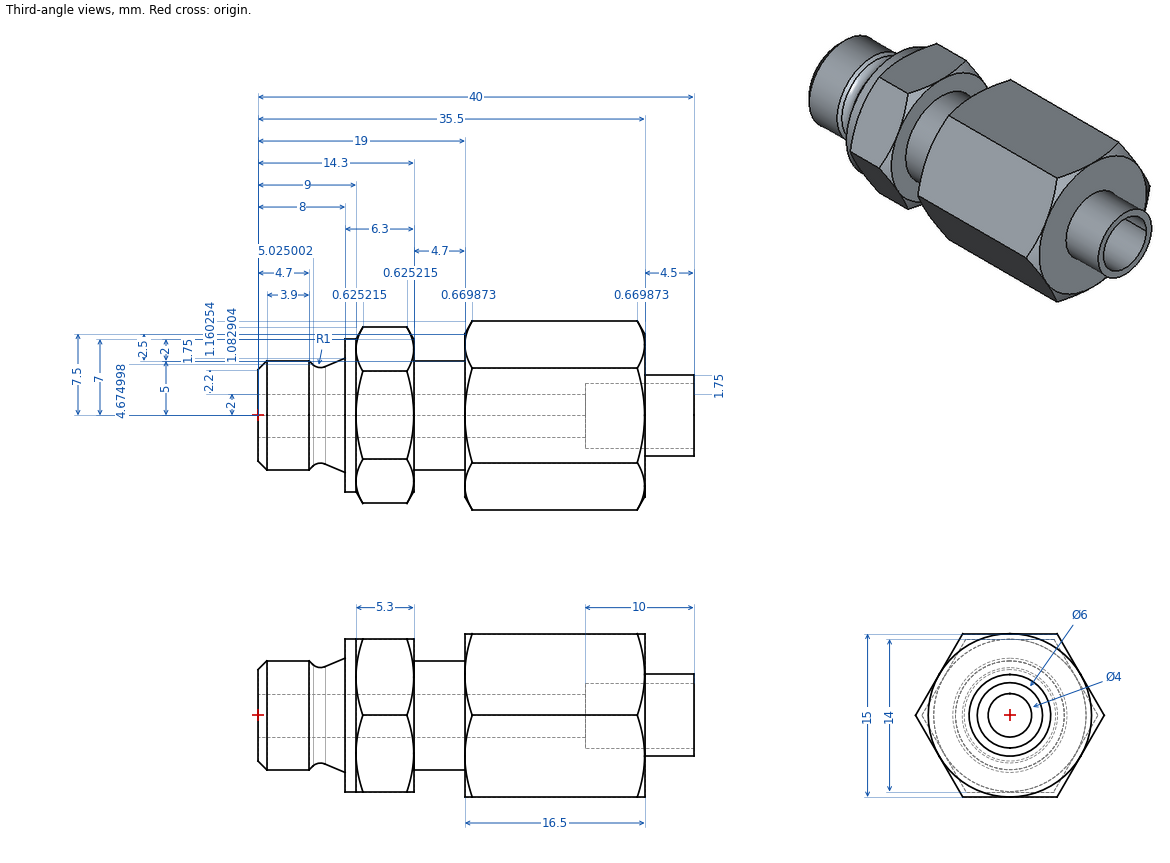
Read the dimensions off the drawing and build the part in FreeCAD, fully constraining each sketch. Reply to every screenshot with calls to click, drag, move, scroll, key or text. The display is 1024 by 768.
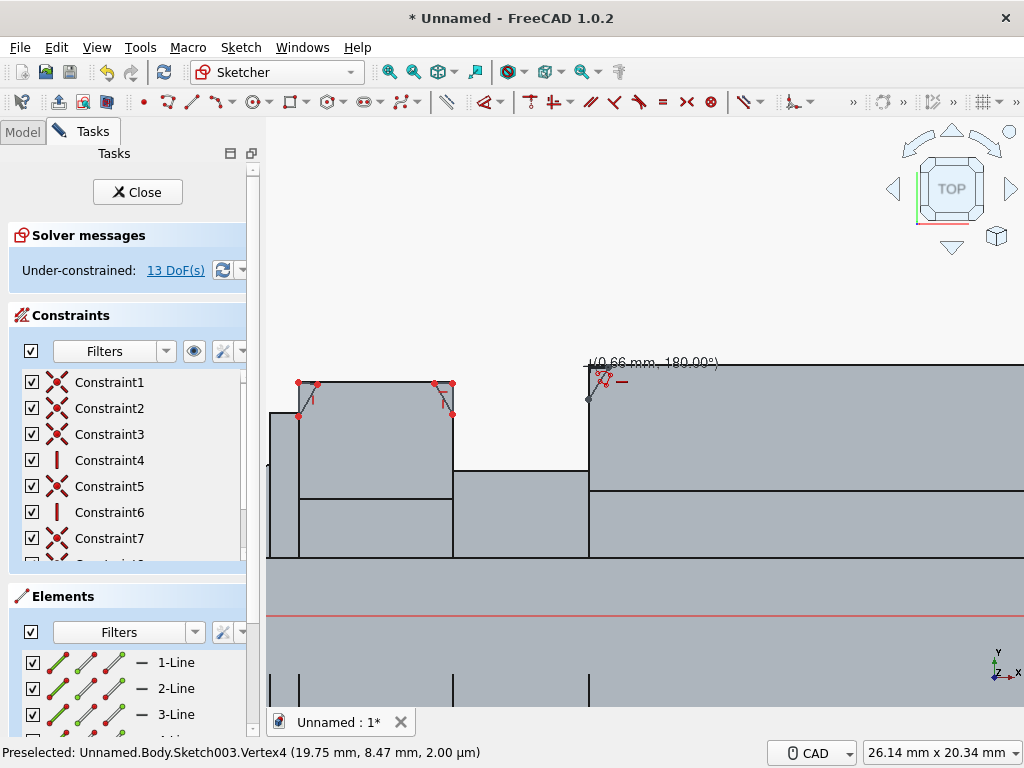
click(589, 365)
click(589, 400)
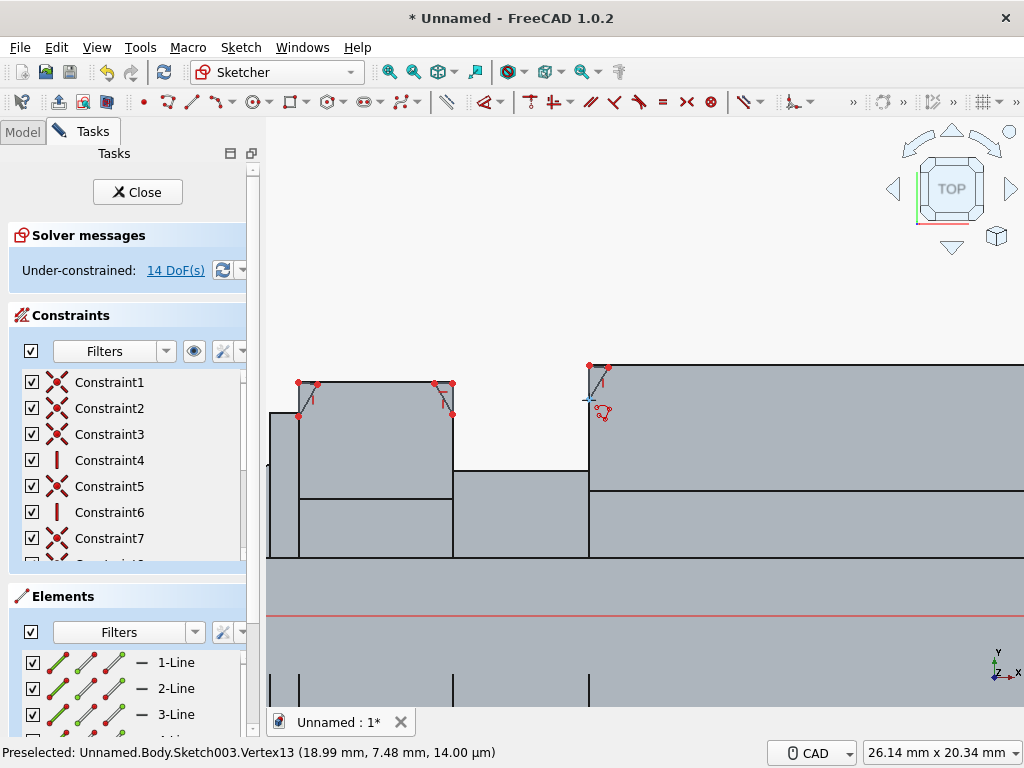
scroll(590, 366, down, 5)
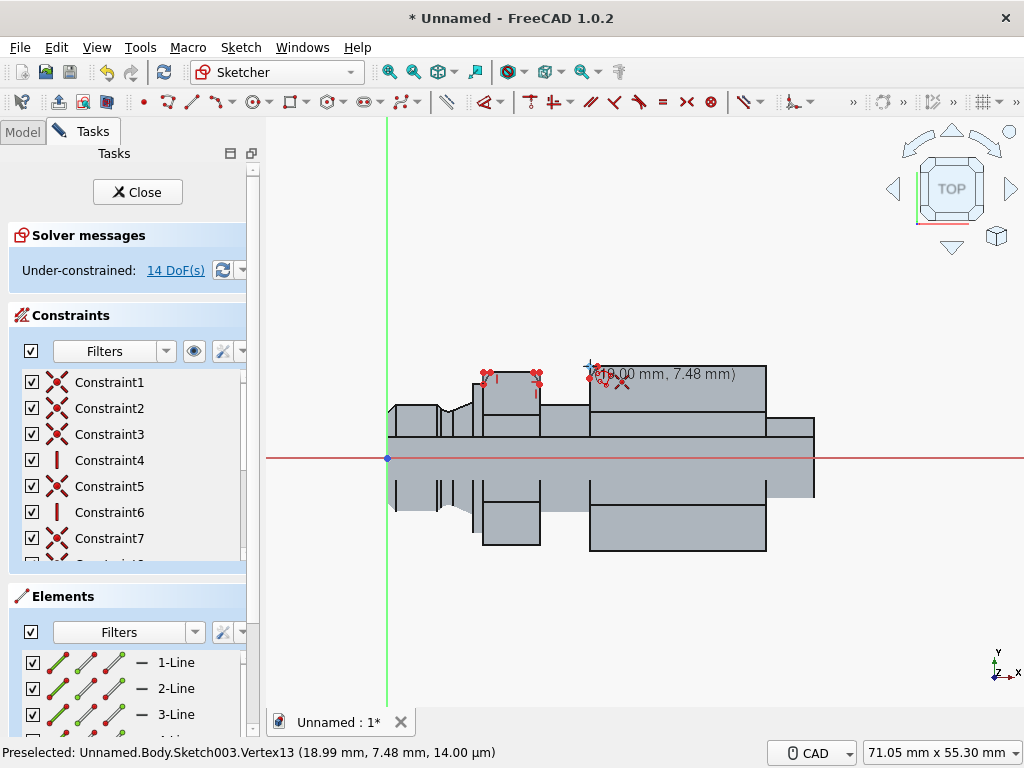
click(759, 366)
click(766, 378)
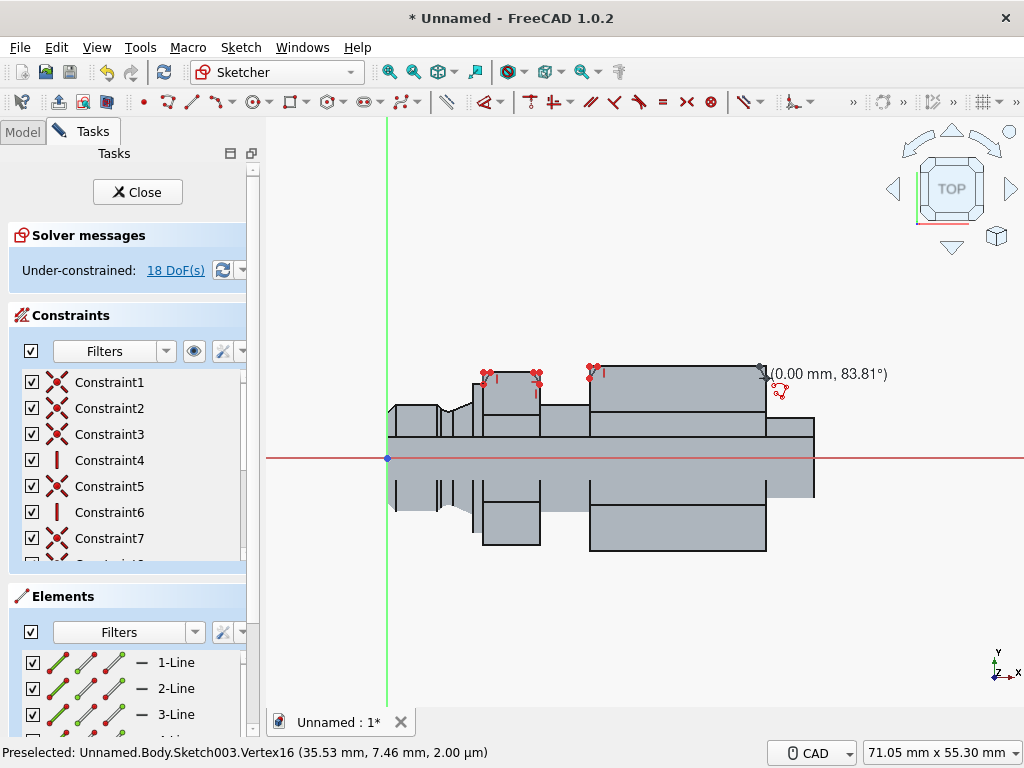
scroll(766, 366, up, 5)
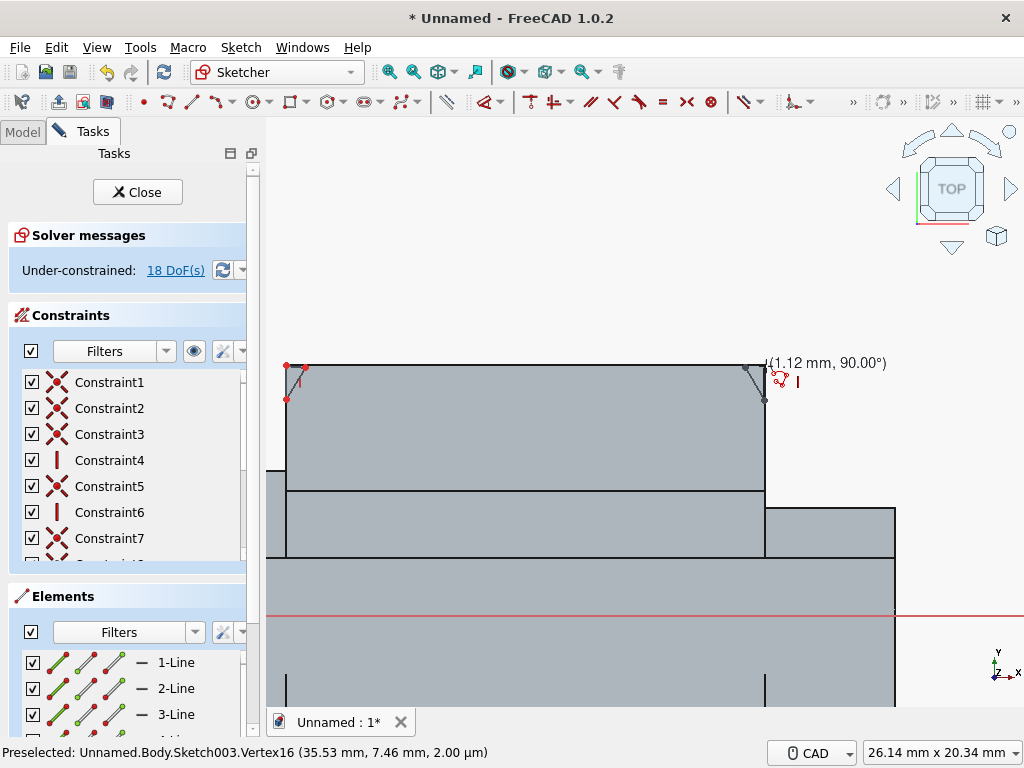
click(765, 365)
click(746, 368)
key(Escape)
key(Escape)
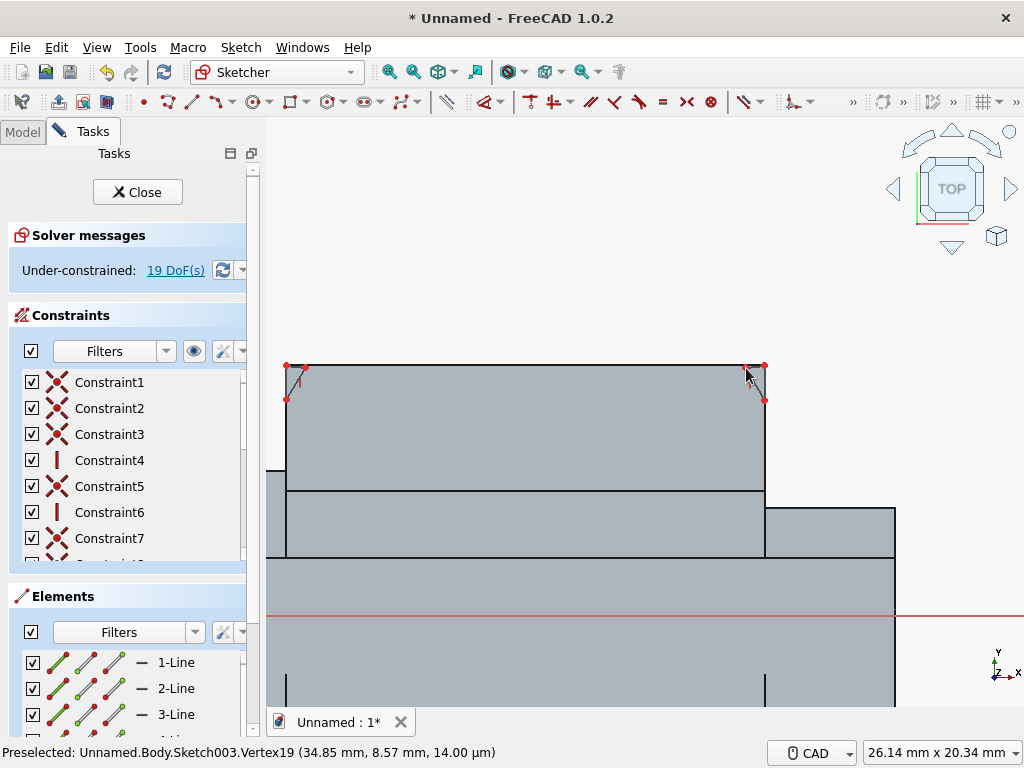
scroll(766, 366, down, 5)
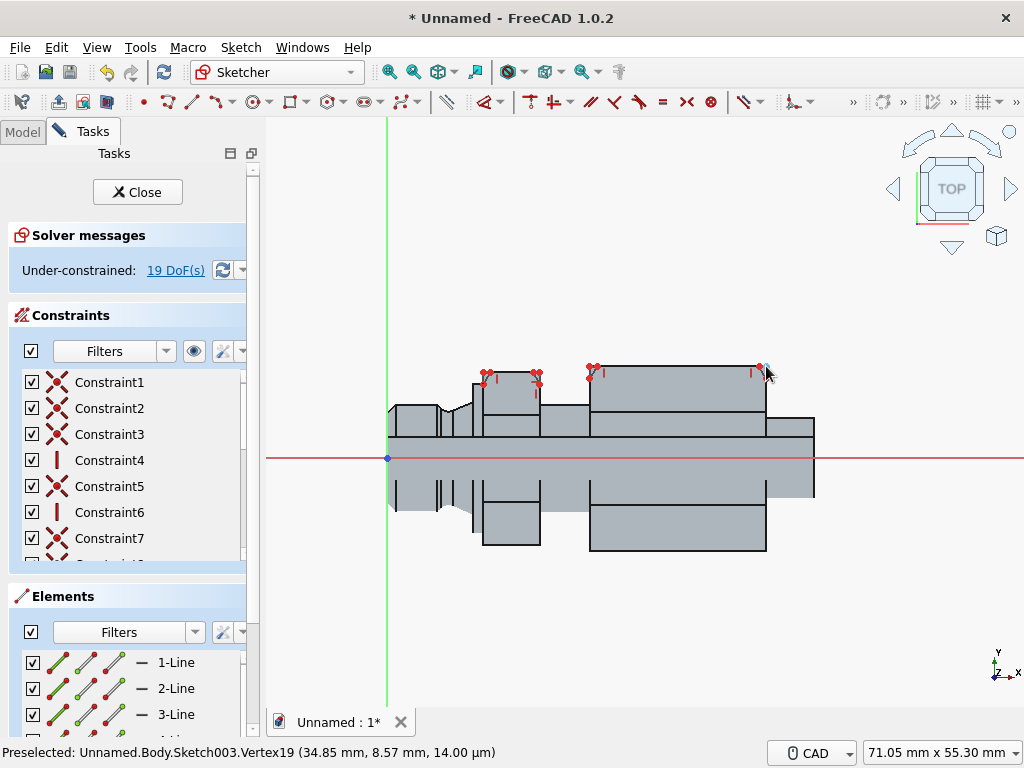
scroll(487, 373, up, 8)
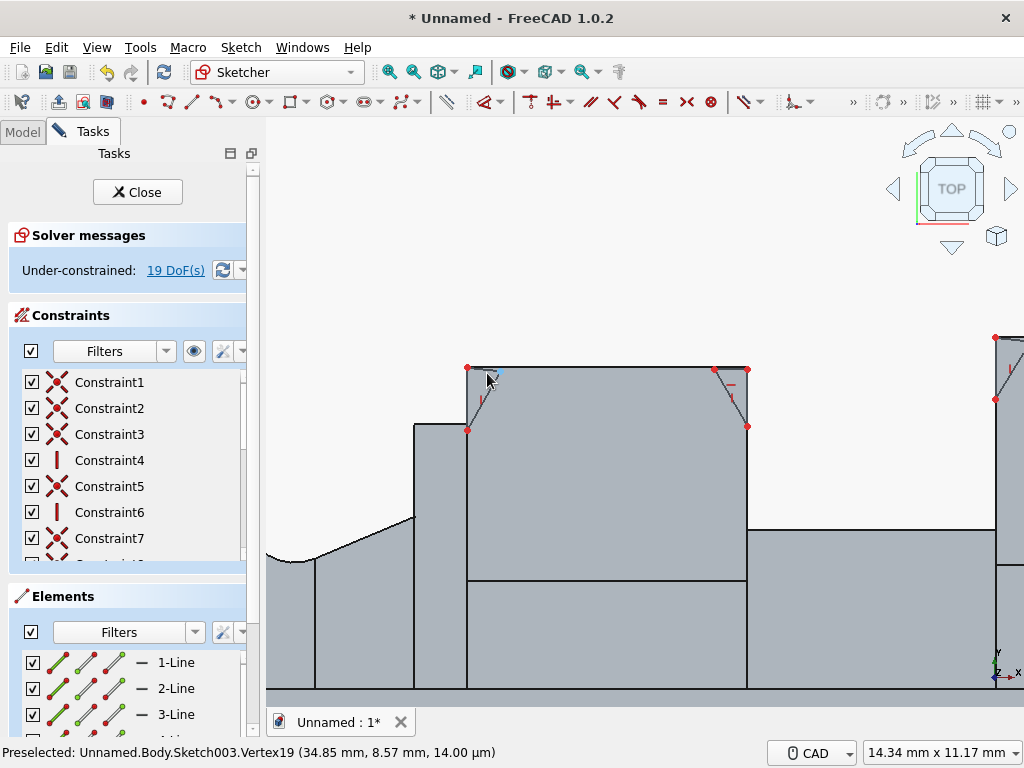
click(484, 370)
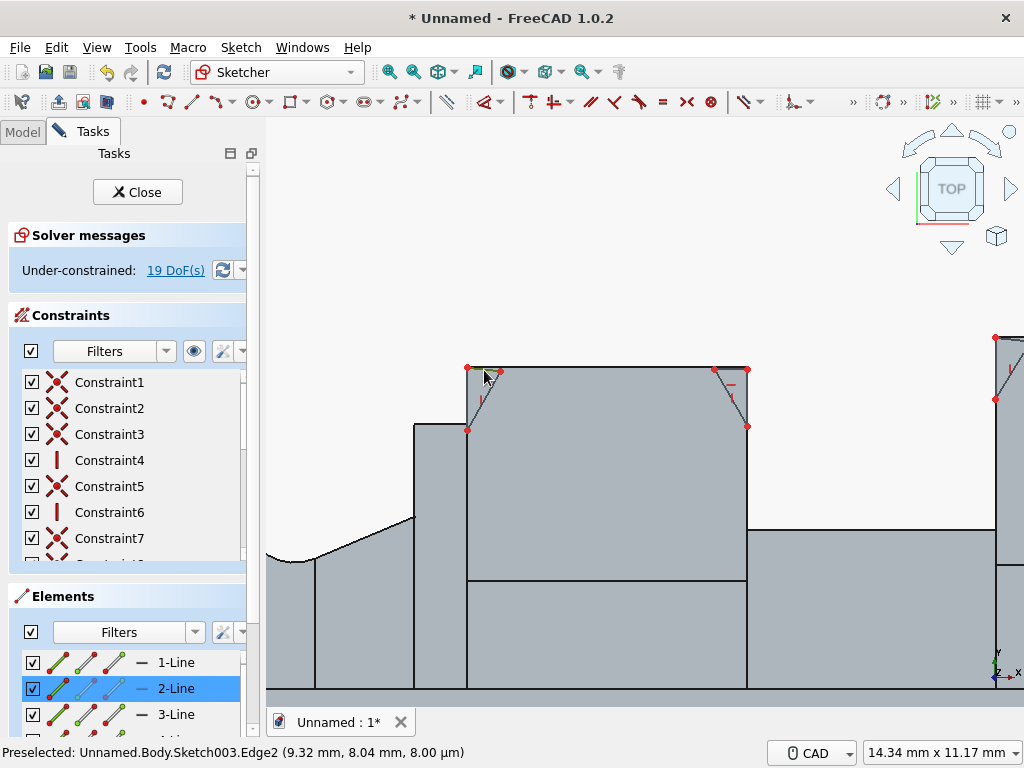
key(h)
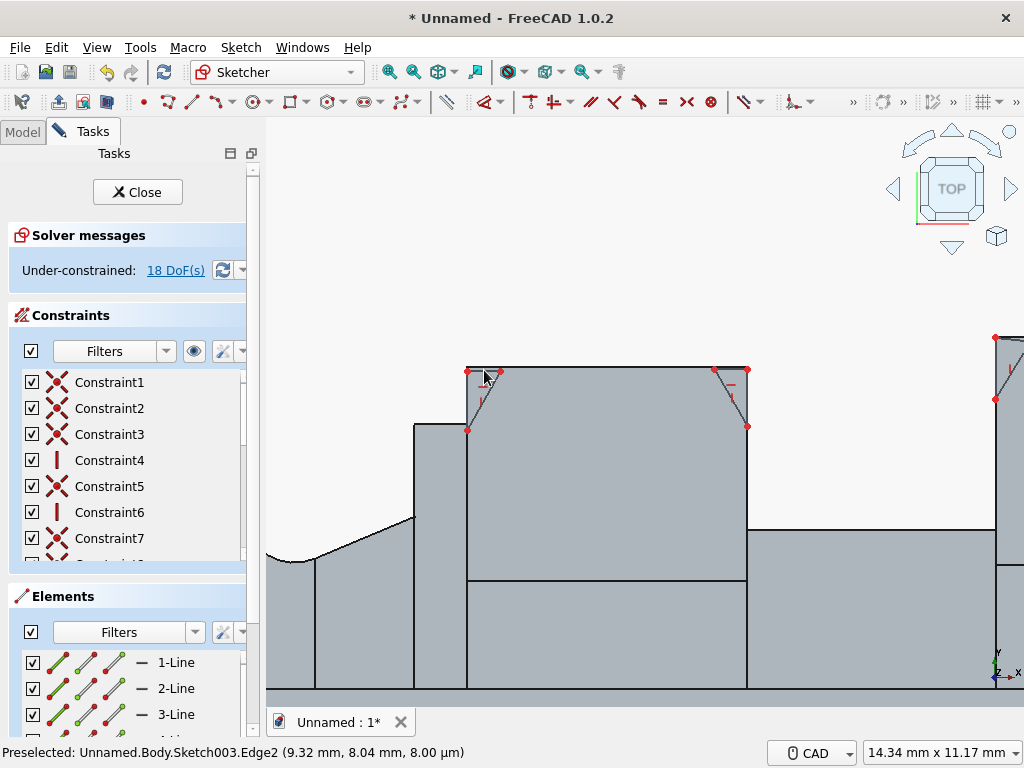
scroll(487, 373, down, 8)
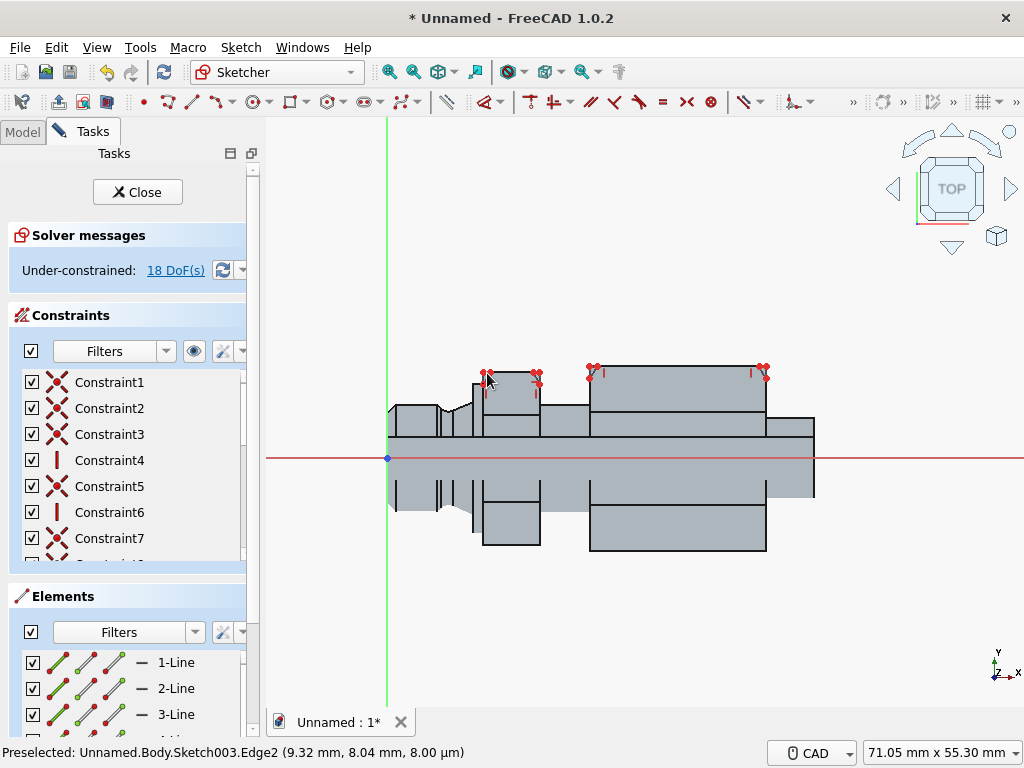
scroll(595, 367, up, 10)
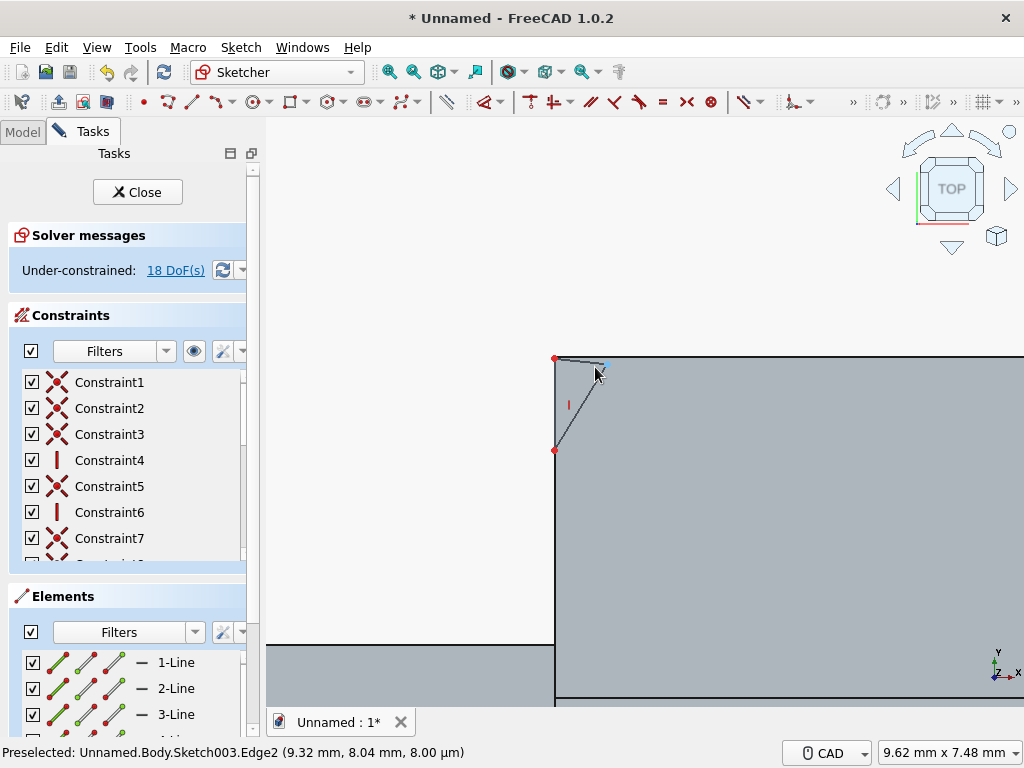
click(591, 363)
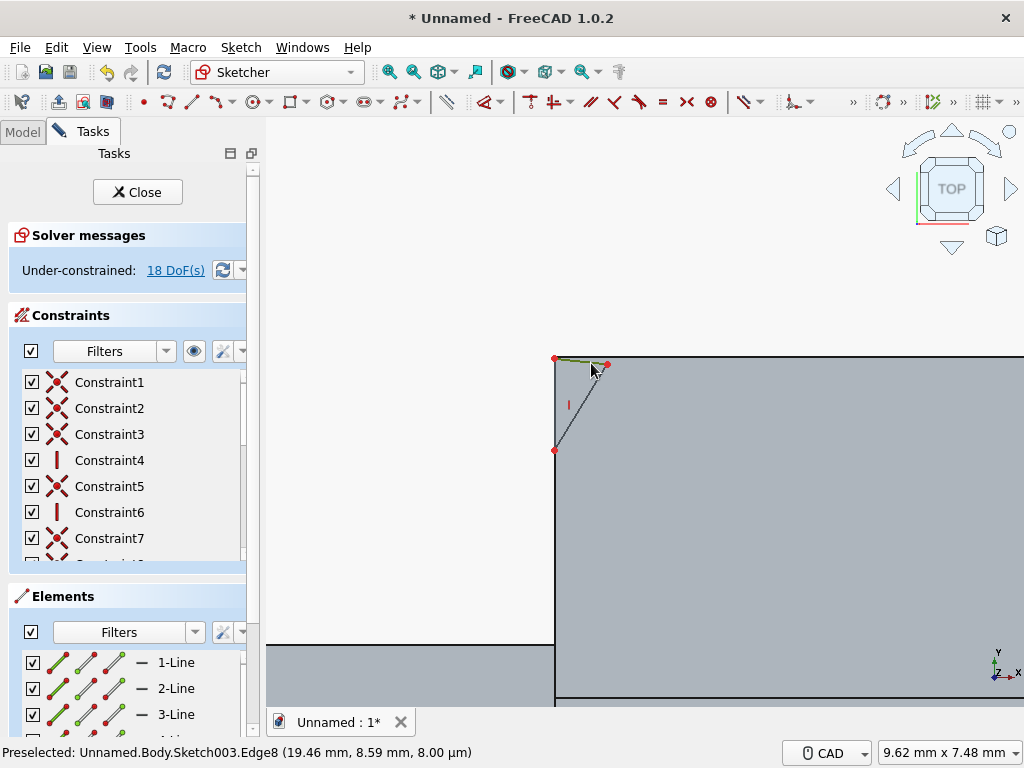
key(h)